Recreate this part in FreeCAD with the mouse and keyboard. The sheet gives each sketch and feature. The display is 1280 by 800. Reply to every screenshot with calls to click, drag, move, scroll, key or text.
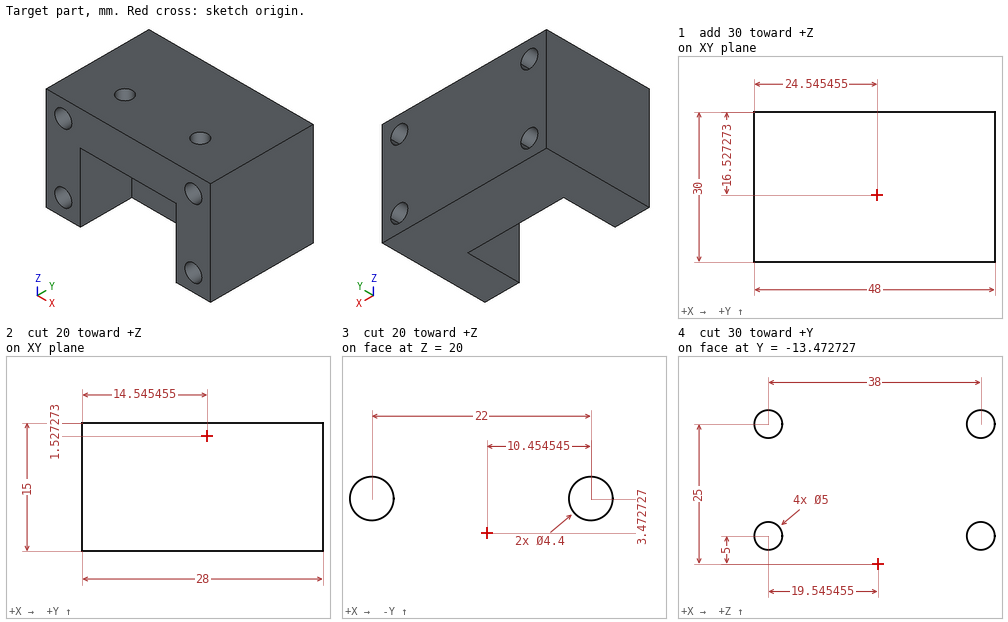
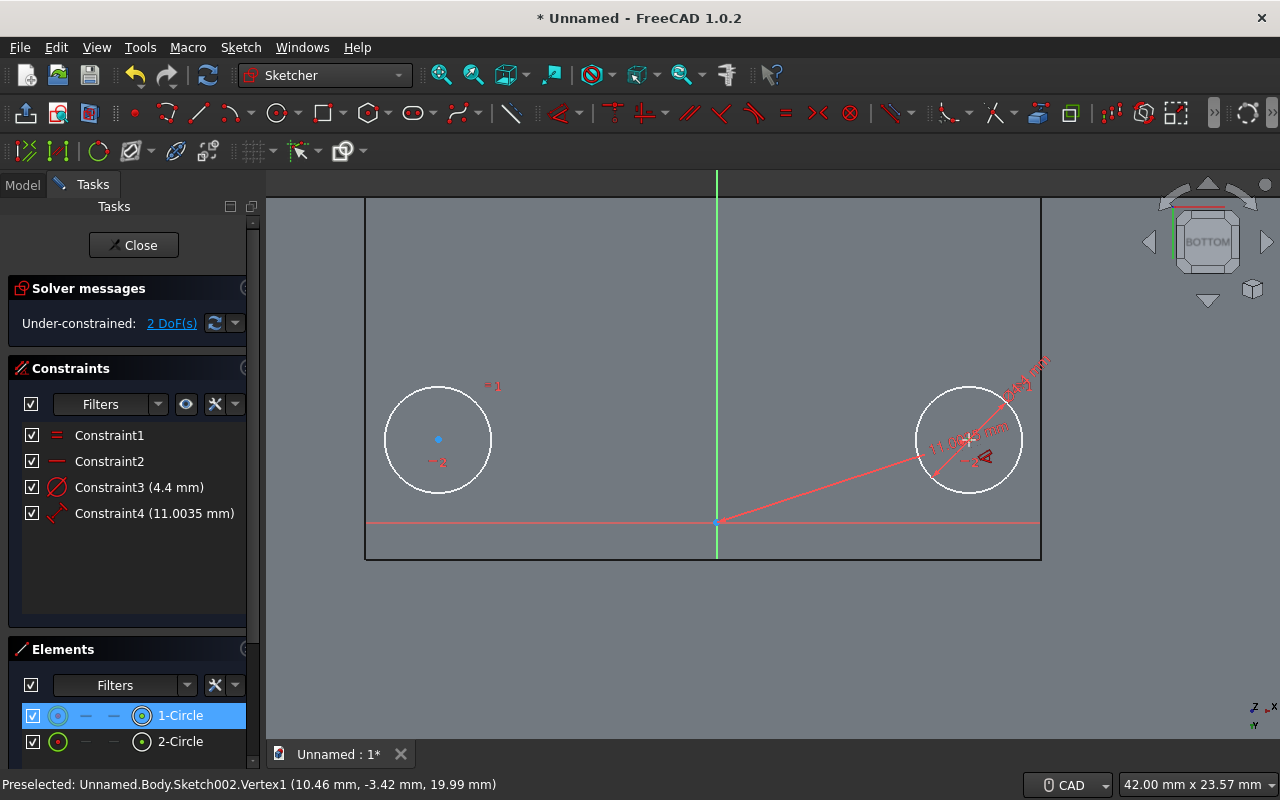
click(438, 440)
click(703, 406)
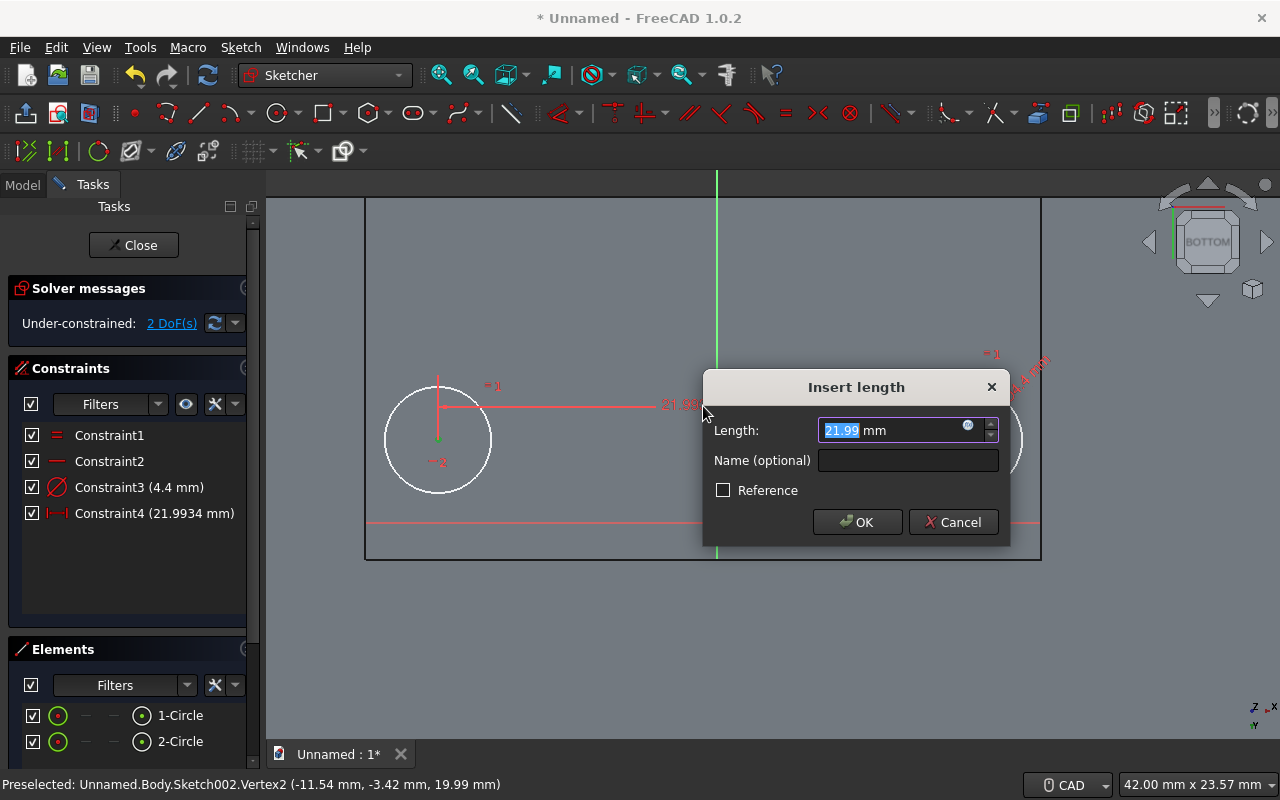
text(22)
key(Return)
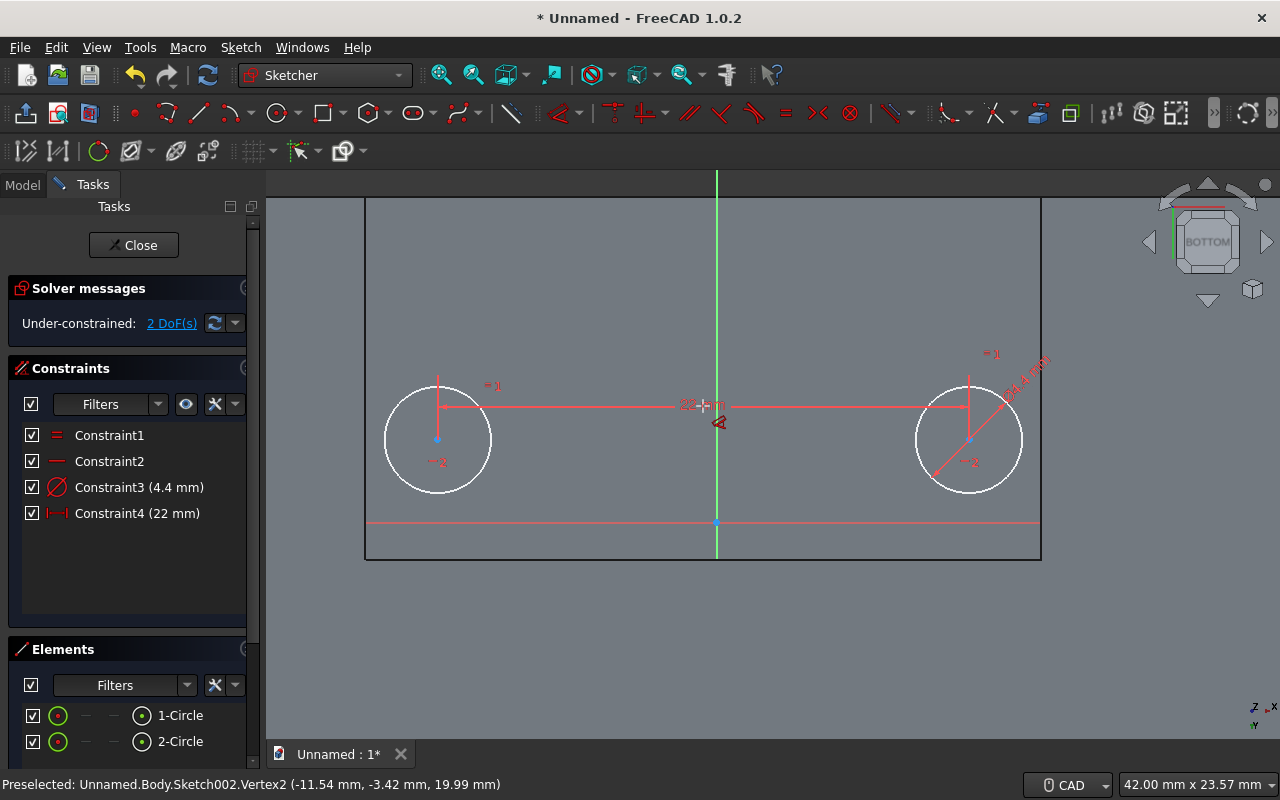
click(969, 440)
click(1003, 500)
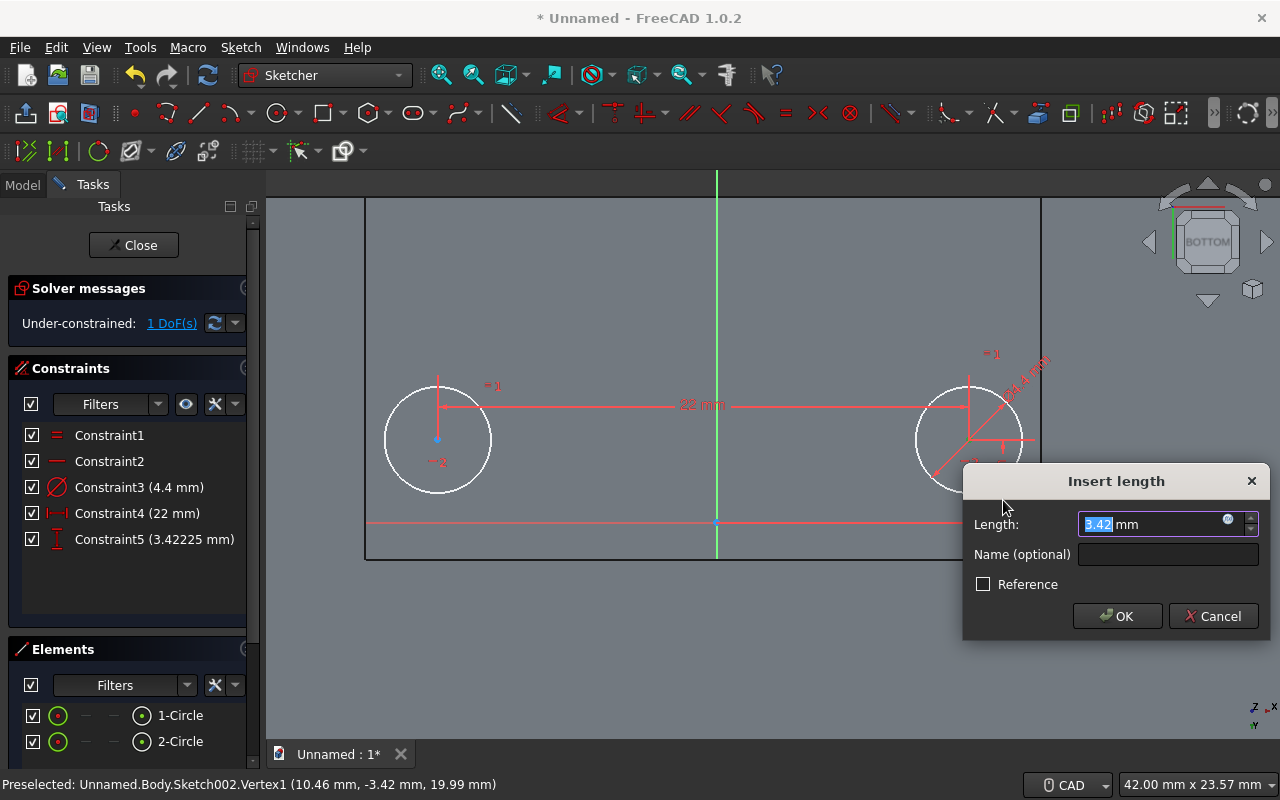
text(3.472727)
key(Return)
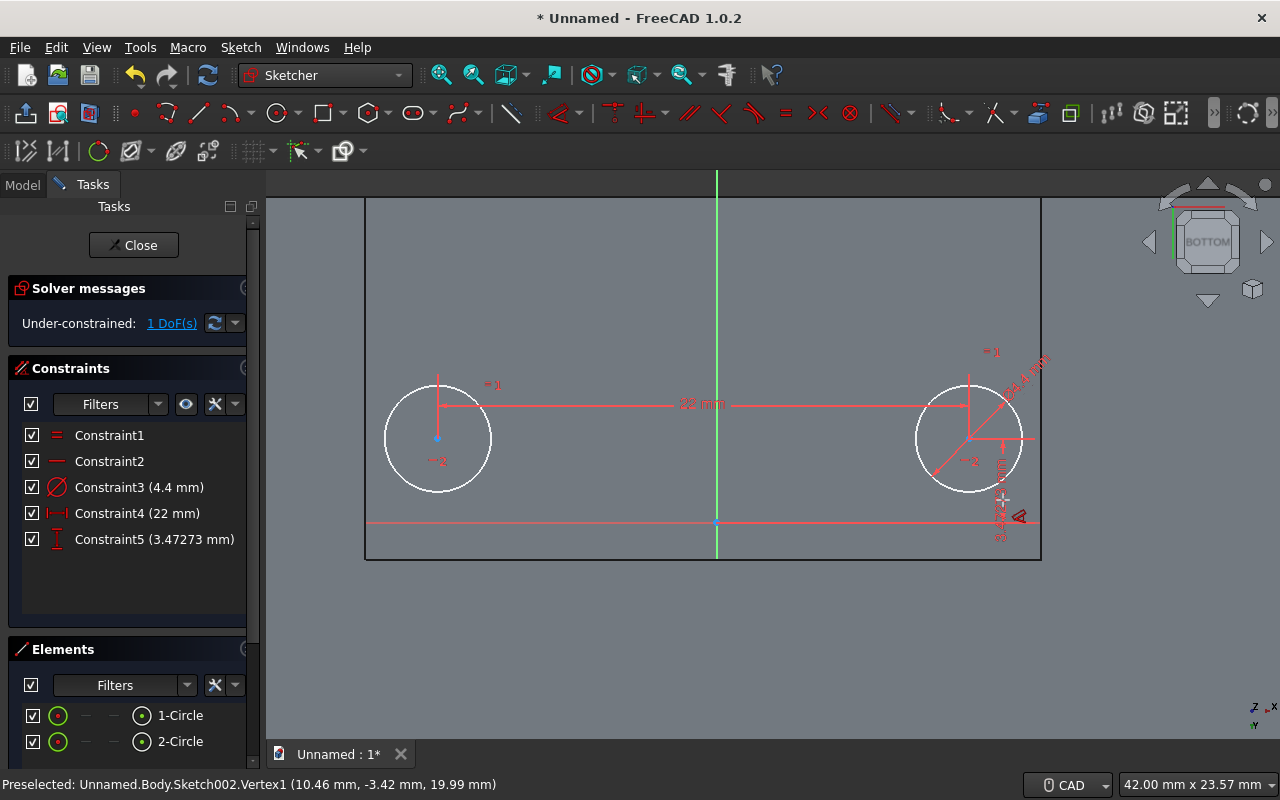
click(969, 439)
click(843, 557)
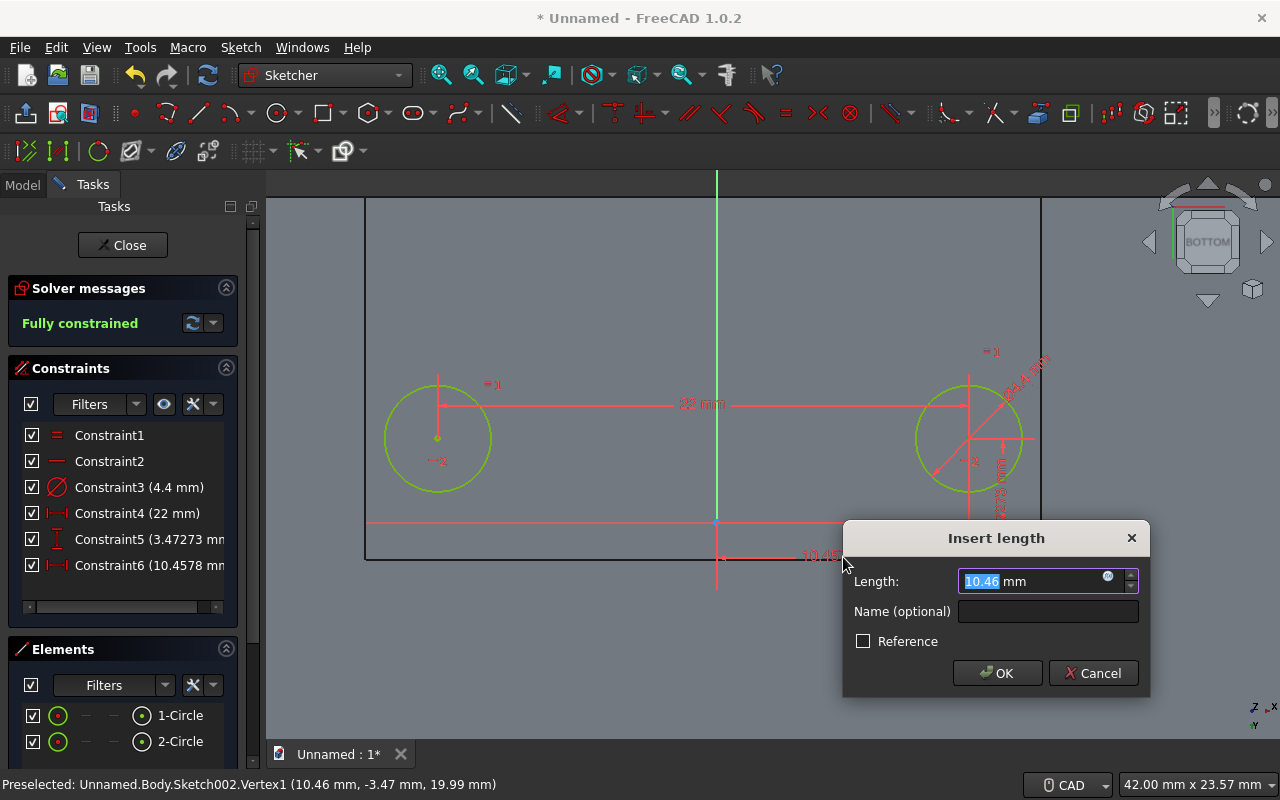
text(10.454545)
key(Return)
key(Escape)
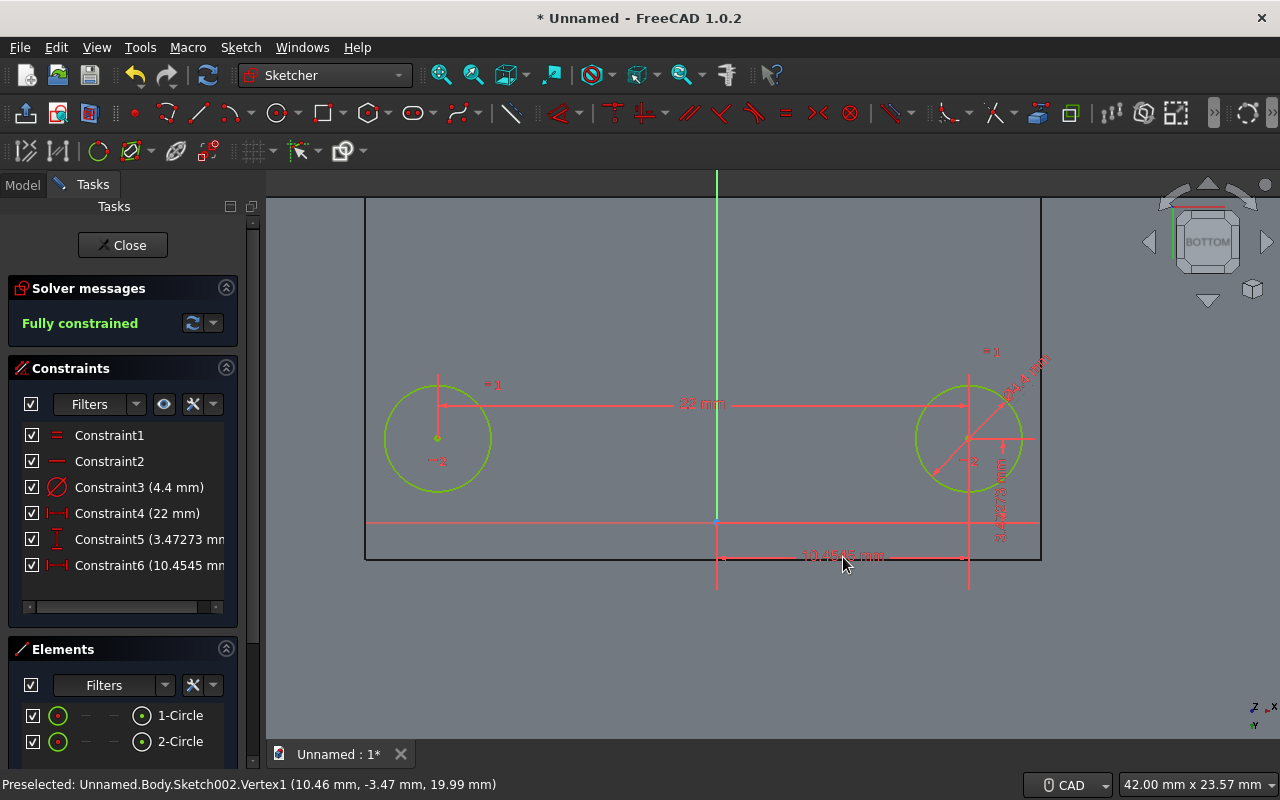
click(123, 245)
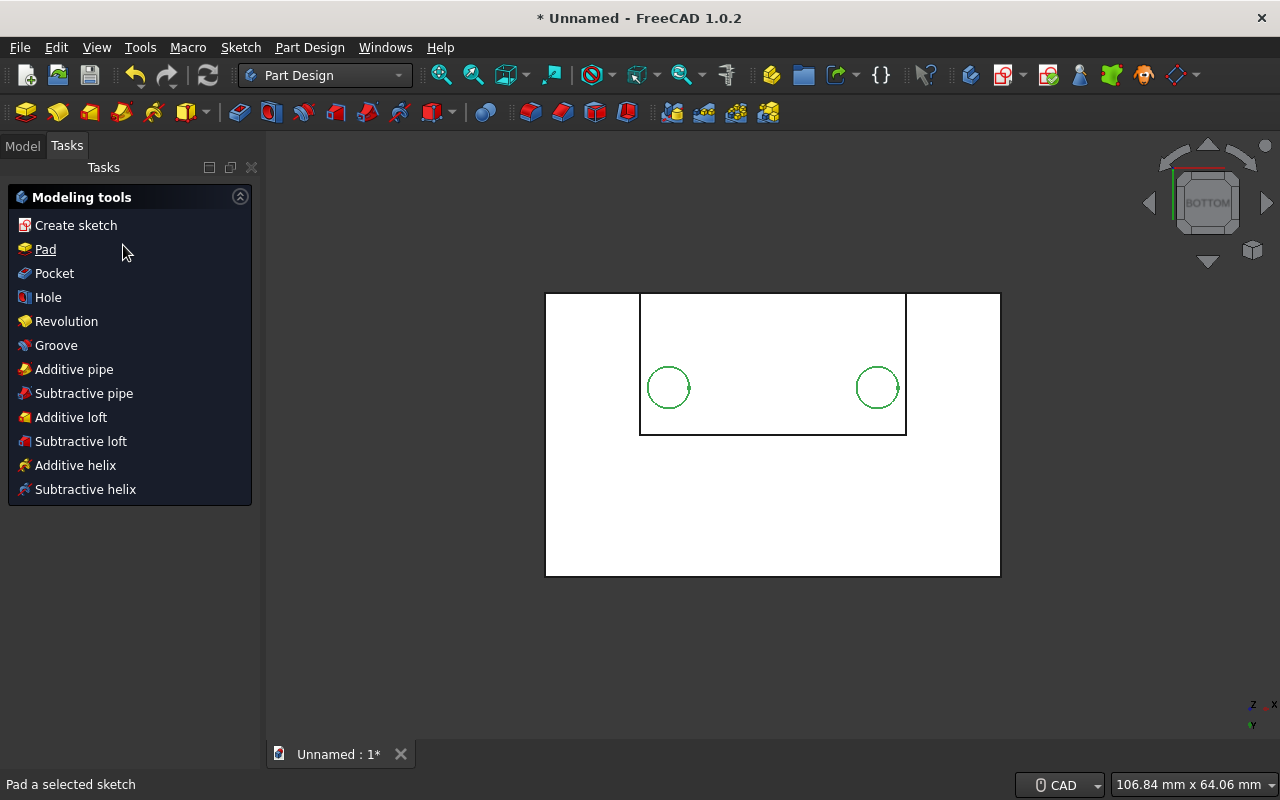
click(240, 112)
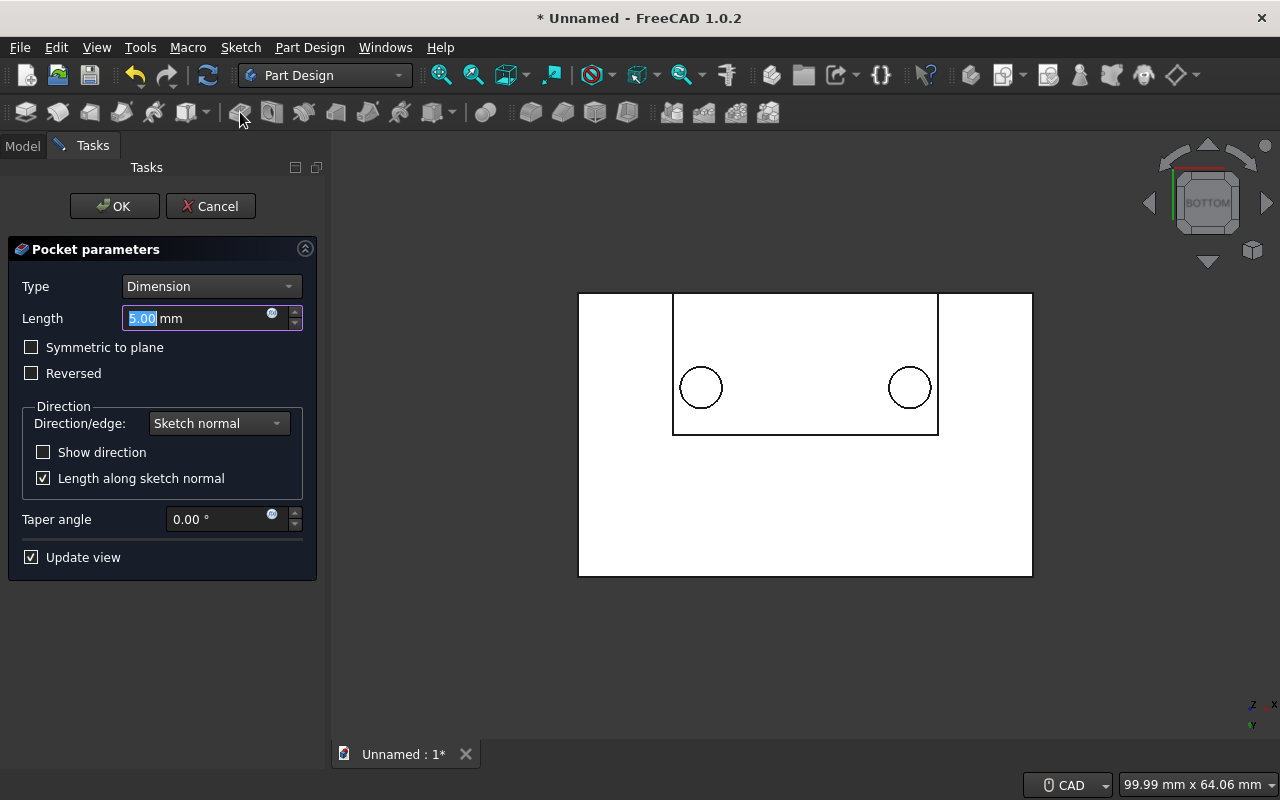
text(20)
key(Tab)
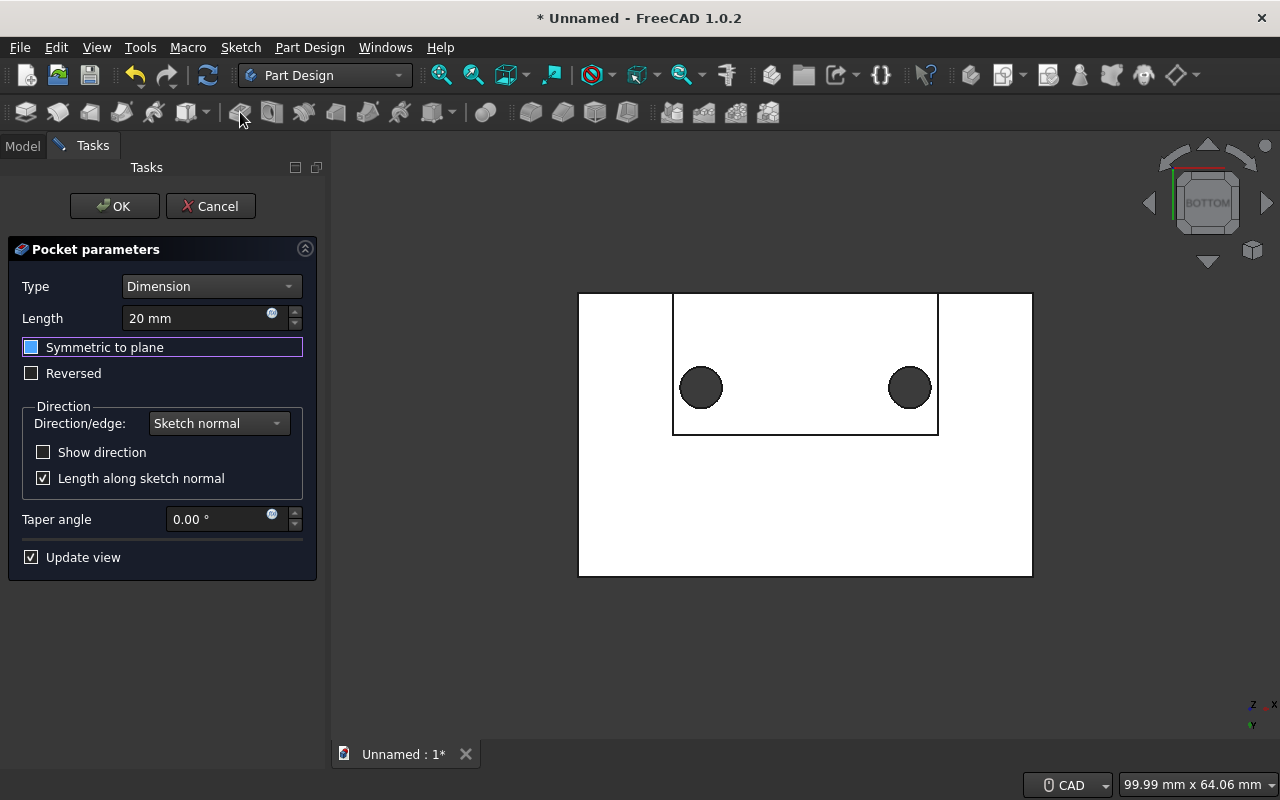
click(115, 206)